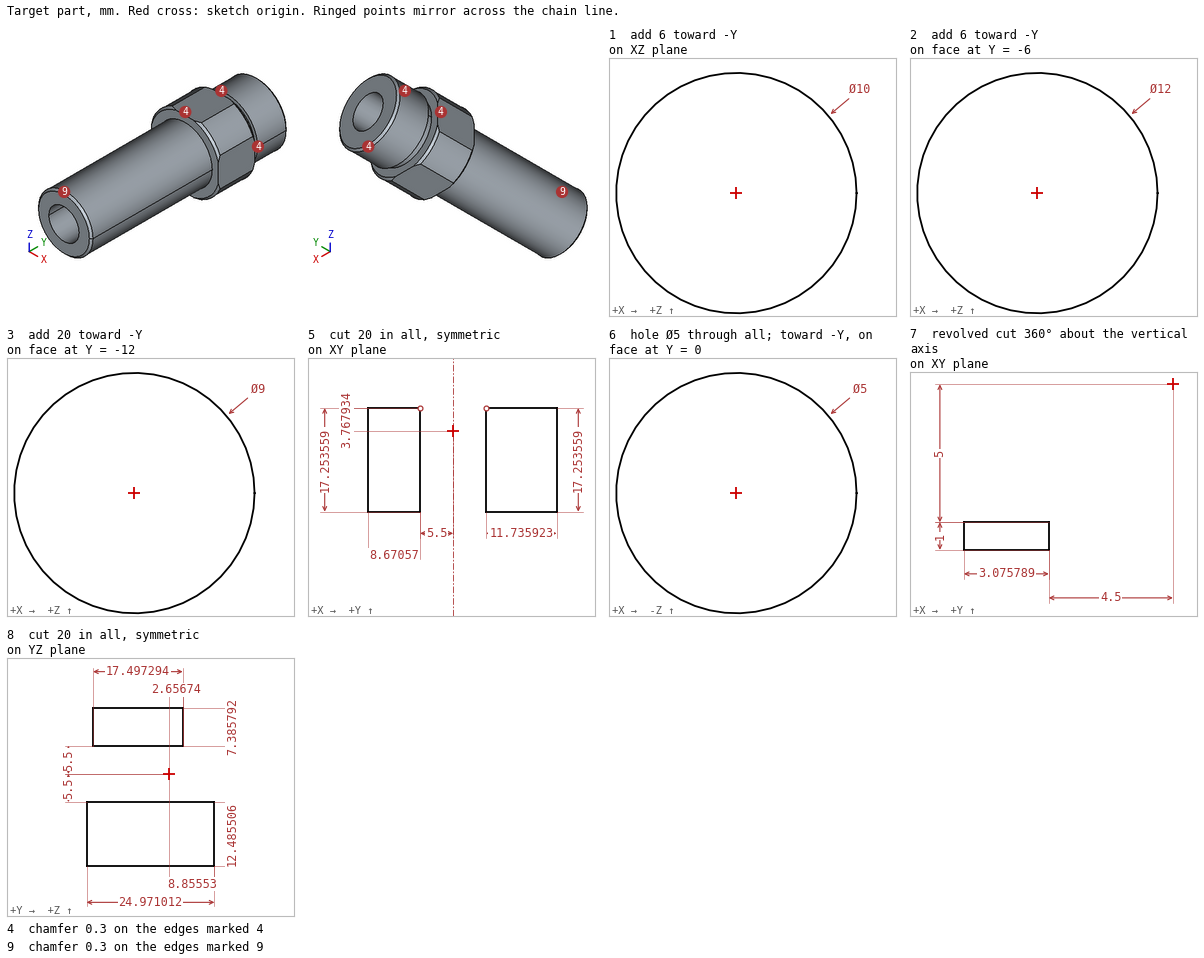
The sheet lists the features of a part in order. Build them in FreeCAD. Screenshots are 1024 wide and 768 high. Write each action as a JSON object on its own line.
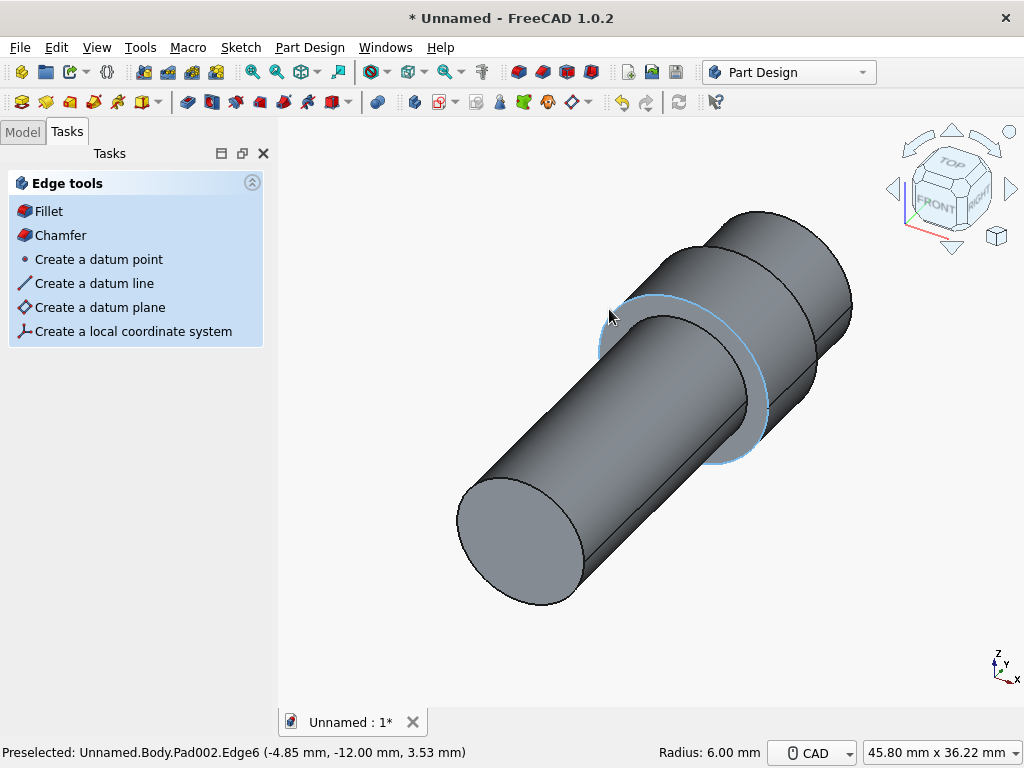
{"action": "key", "text": "0"}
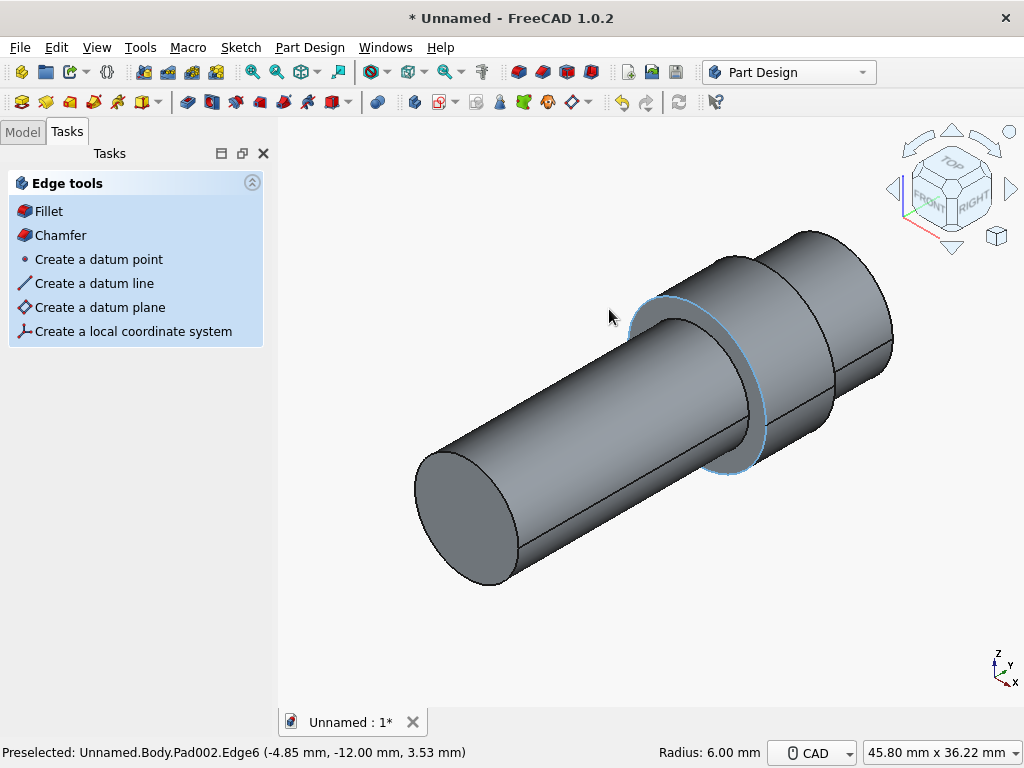
{"action": "key", "text": "2"}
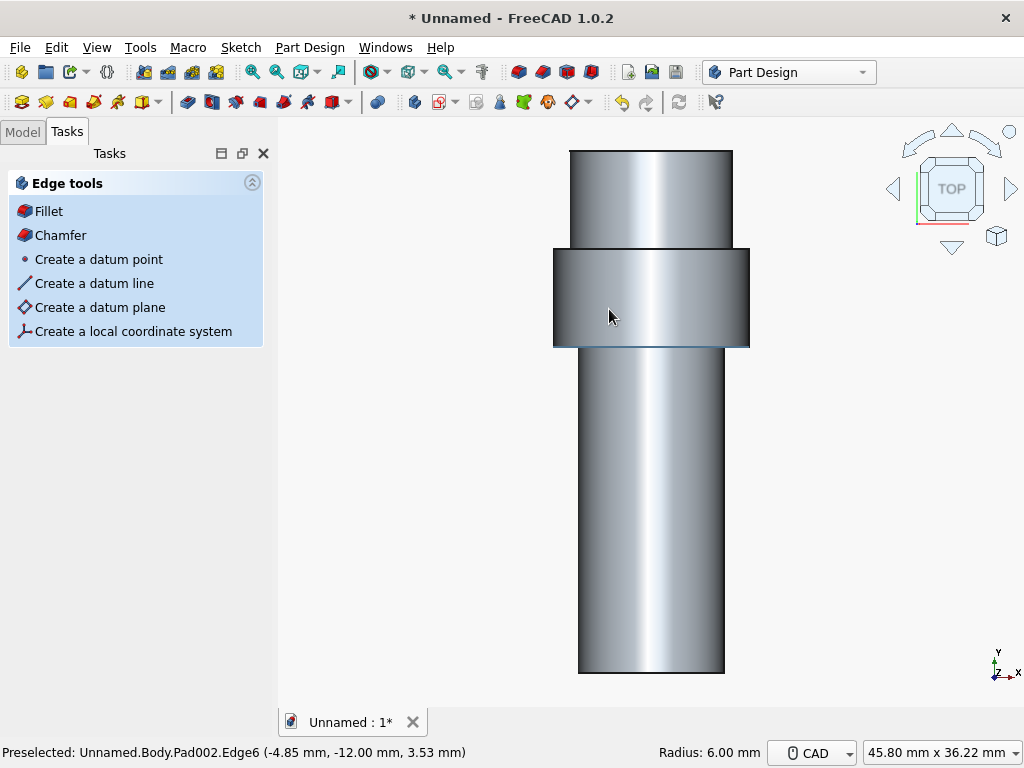
{"action": "left_click", "coordinate": [585, 150], "text": "ctrl"}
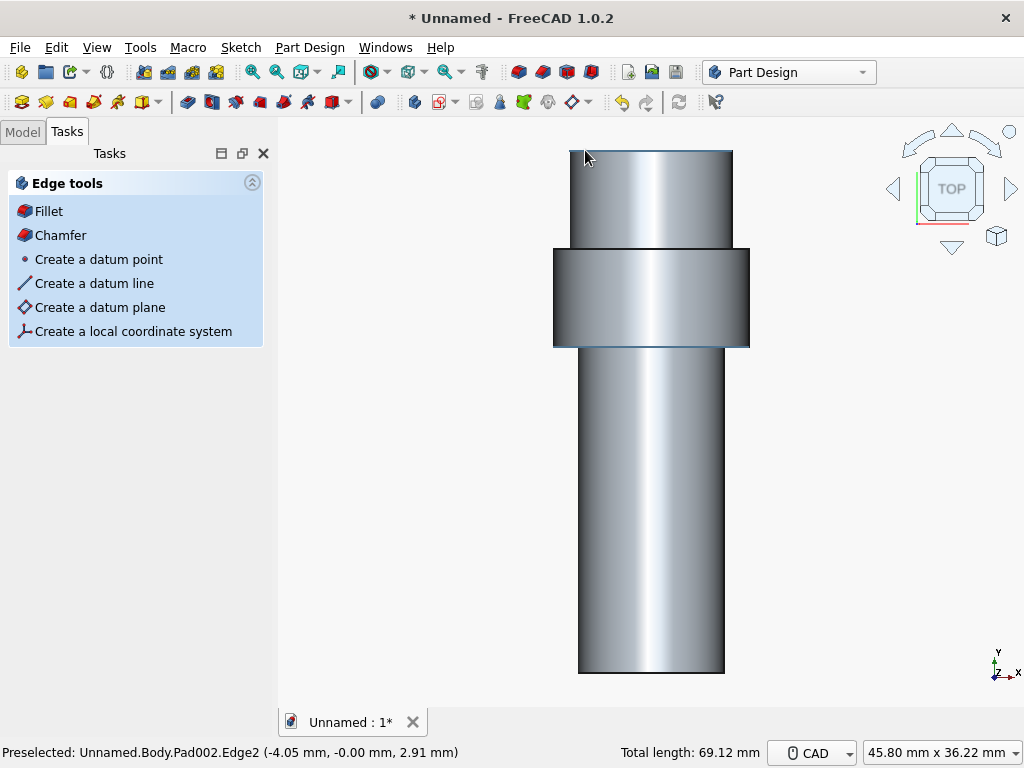
{"action": "left_click", "coordinate": [572, 248], "text": "ctrl"}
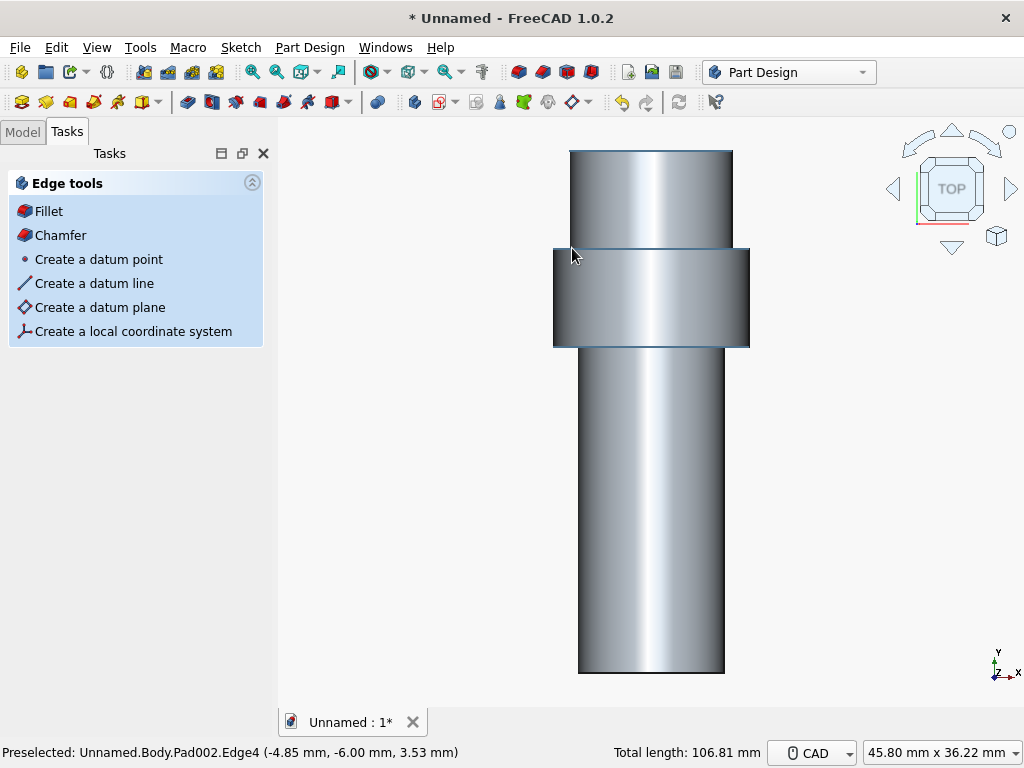
{"action": "left_click", "coordinate": [544, 72]}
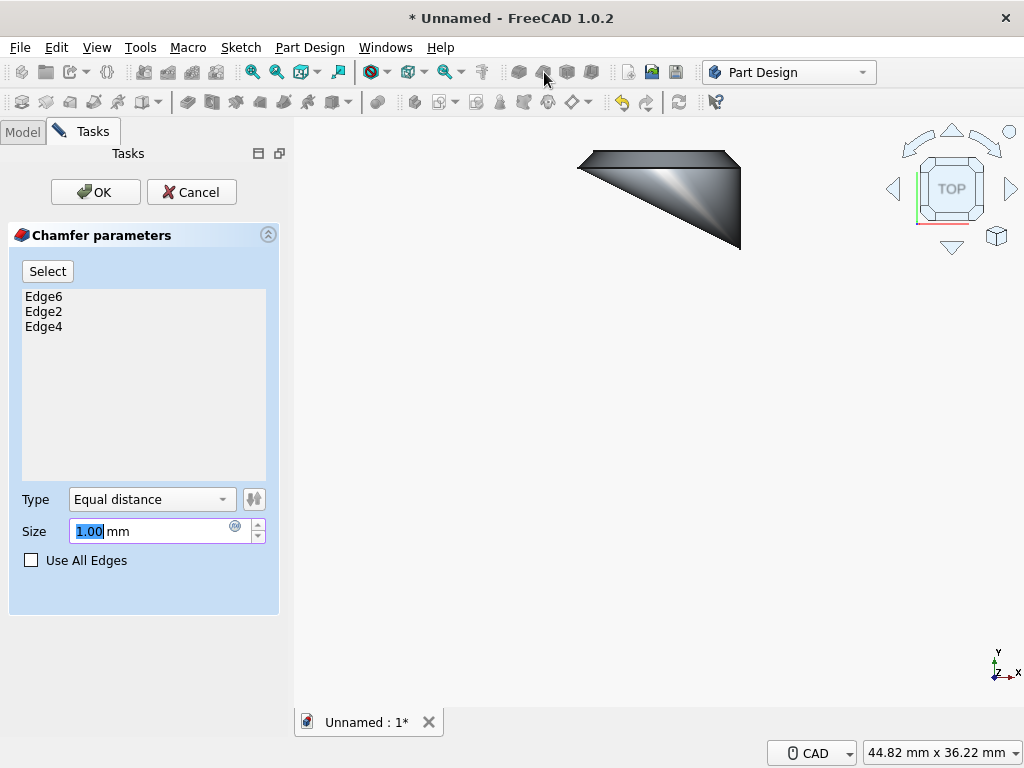
{"action": "type", "text": "0.3"}
{"action": "key", "text": "Tab"}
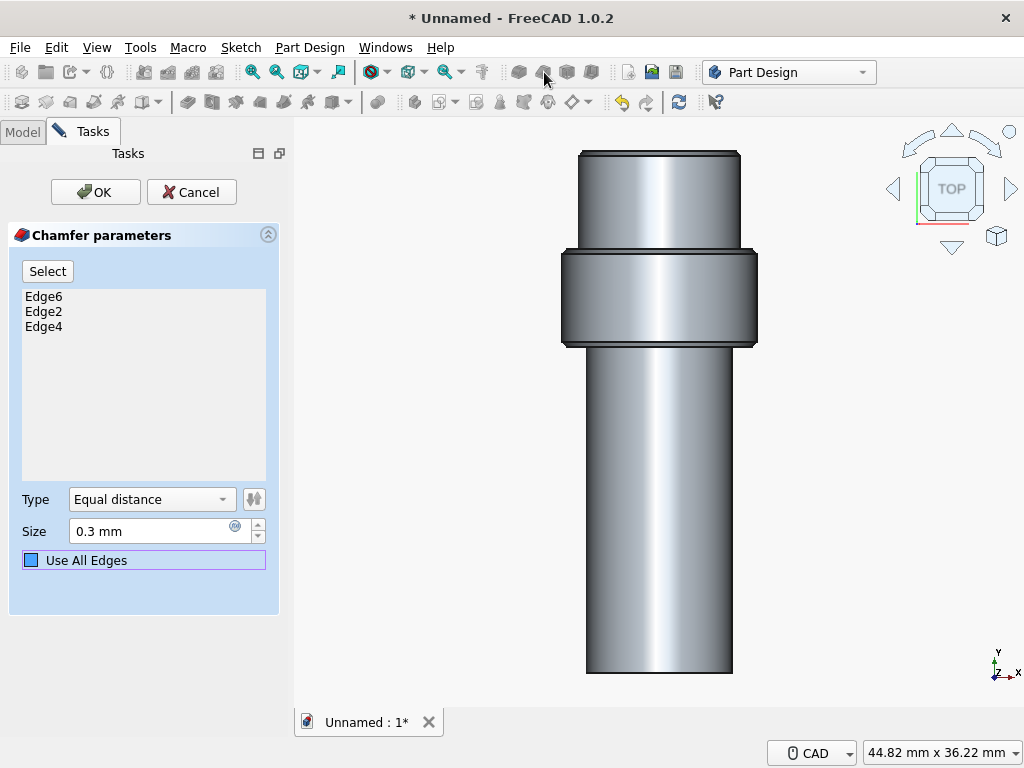
{"action": "left_click", "coordinate": [96, 192]}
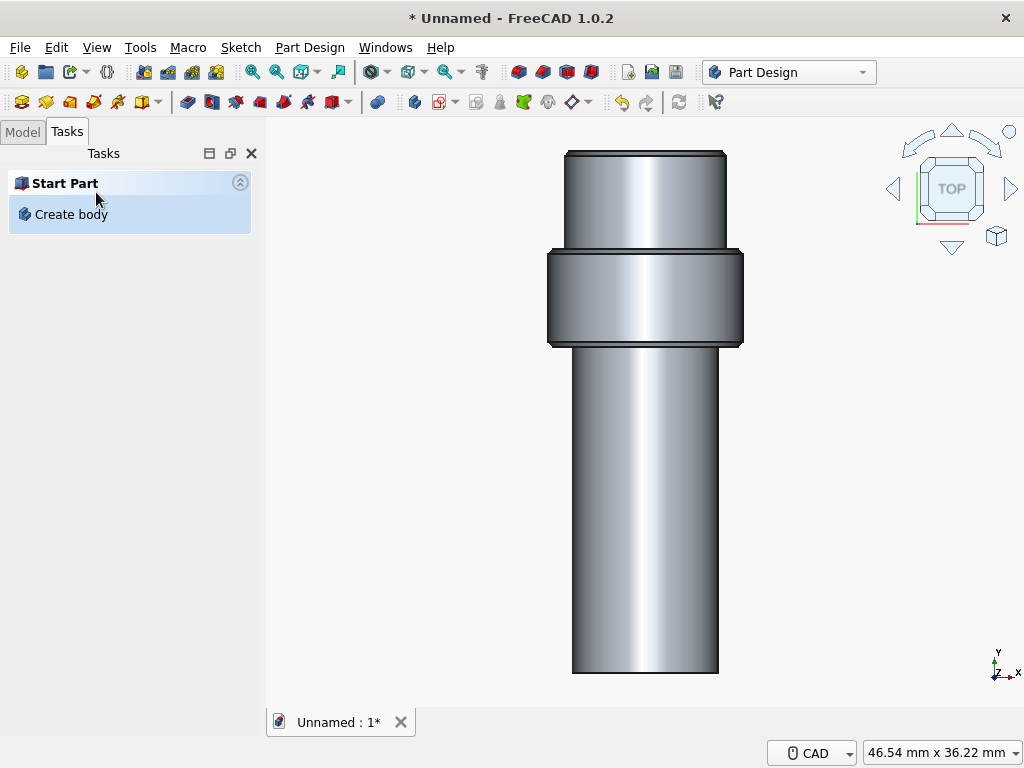
{"action": "left_click", "coordinate": [440, 102]}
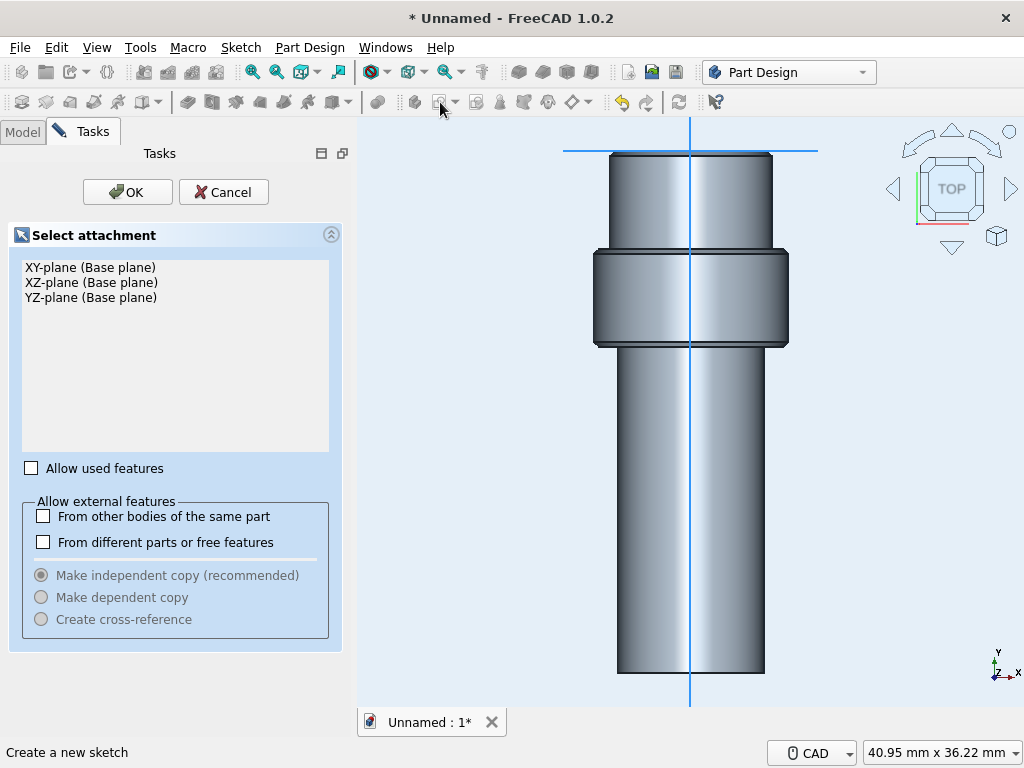
{"action": "left_click", "coordinate": [82, 268]}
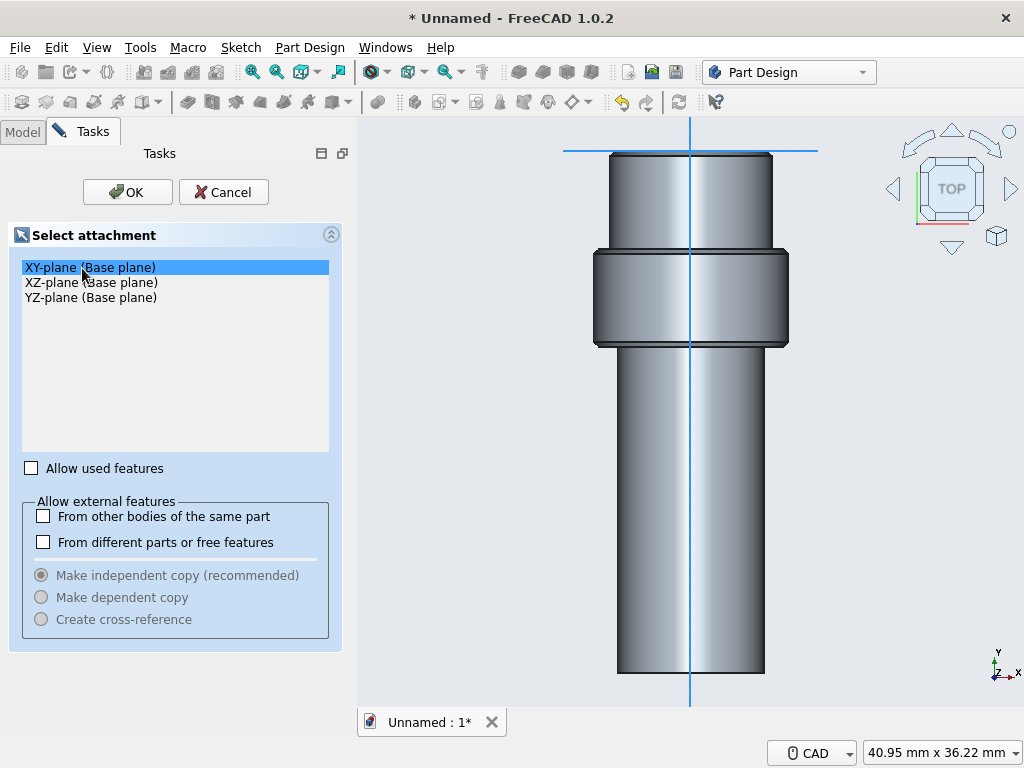
{"action": "left_click", "coordinate": [128, 192]}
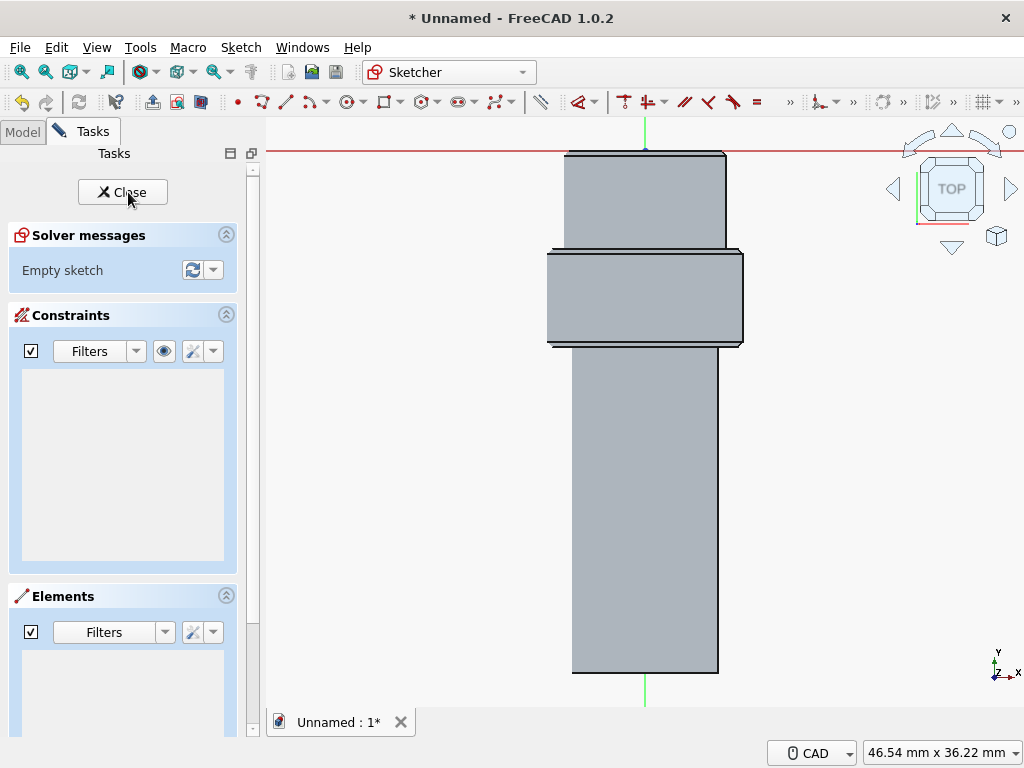
{"action": "key", "text": "q s"}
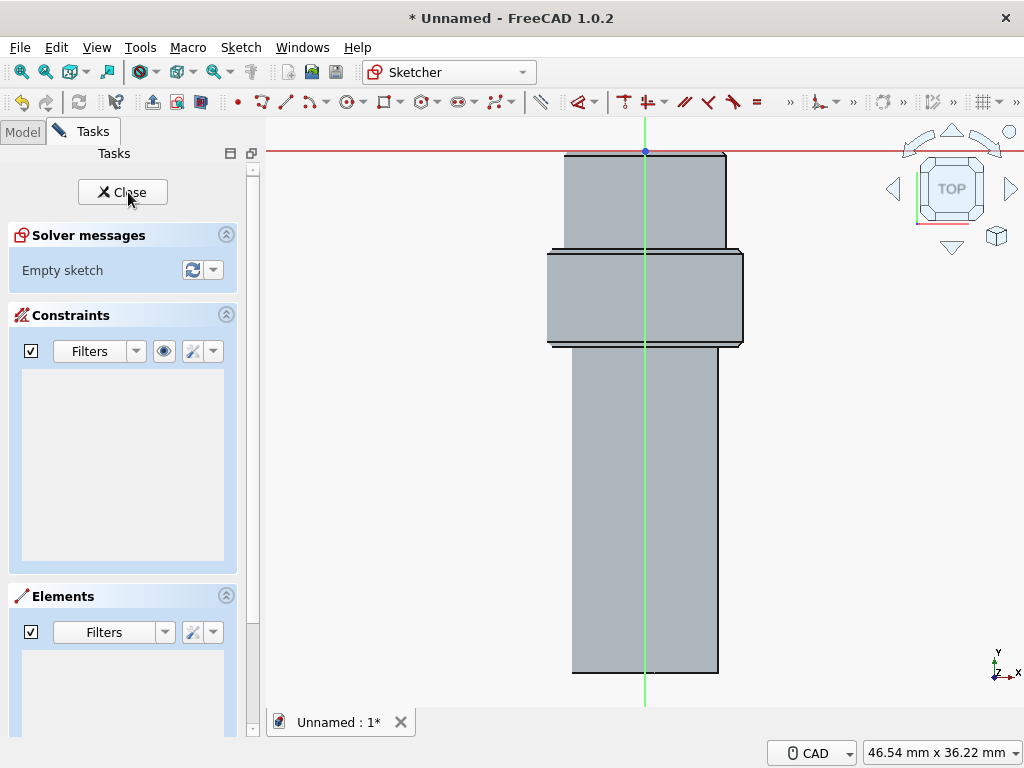
{"action": "scroll", "coordinate": [294, 679], "scroll_direction": "down", "scroll_amount": 1}